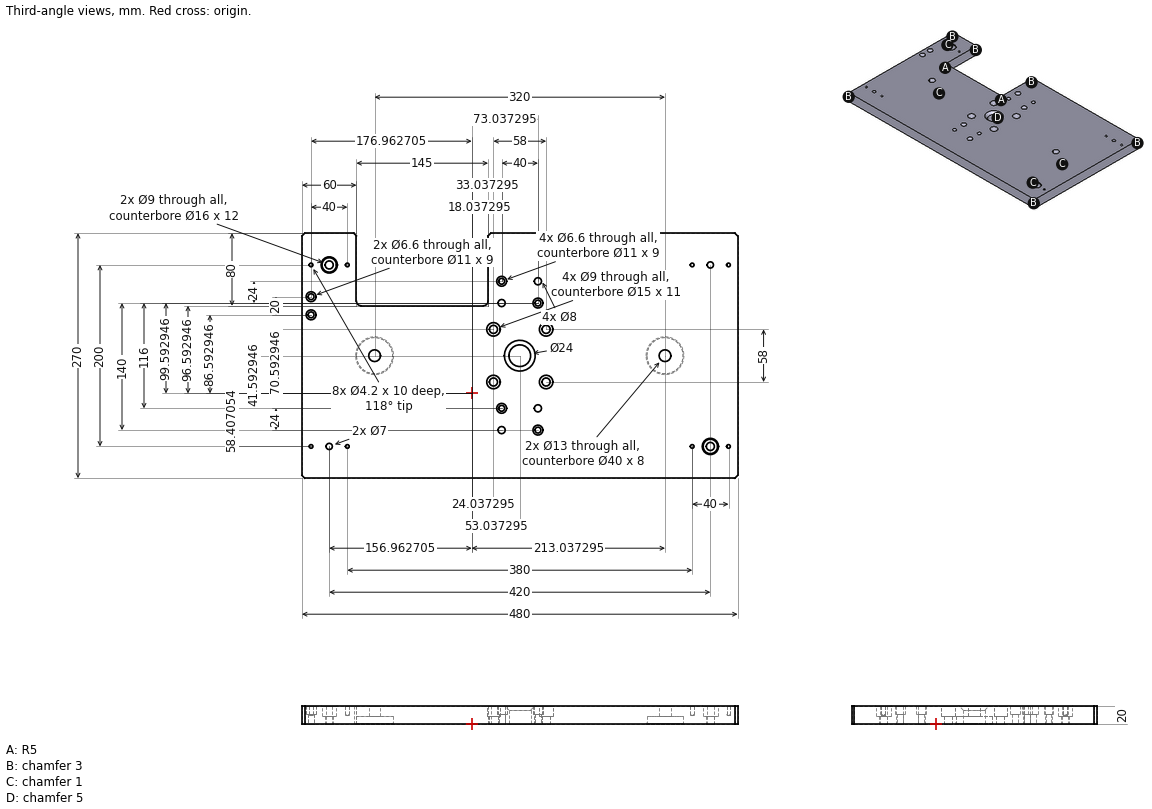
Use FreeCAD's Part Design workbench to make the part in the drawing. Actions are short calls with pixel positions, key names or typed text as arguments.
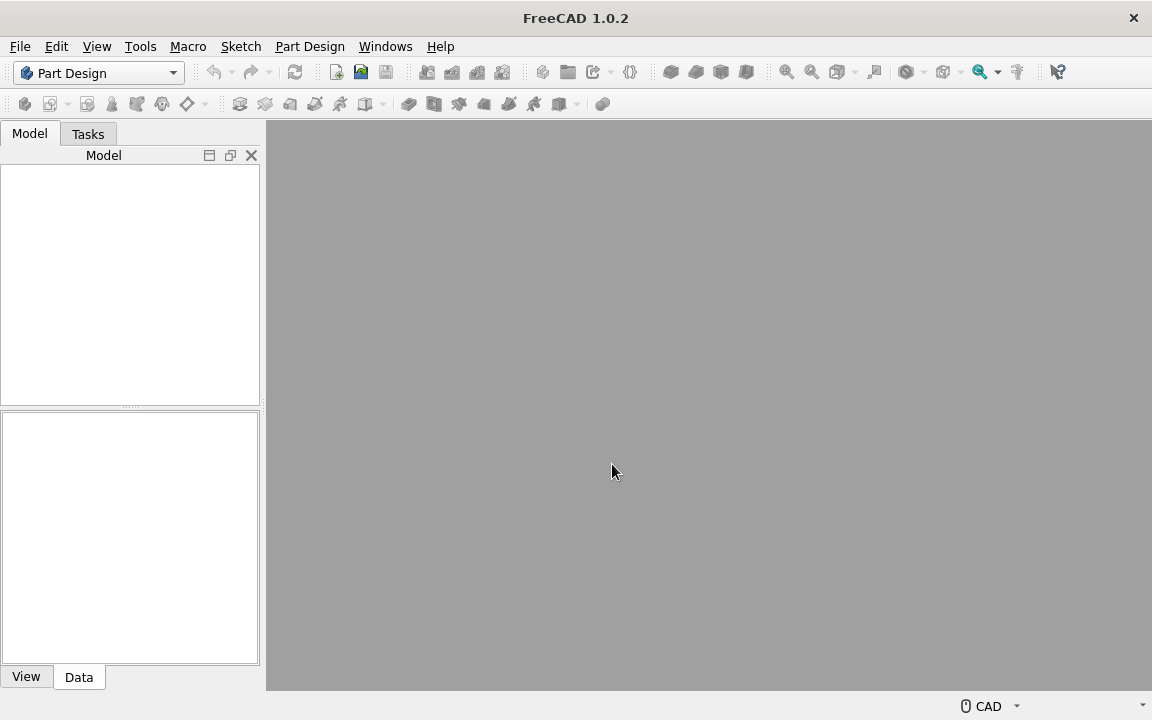
click(336, 72)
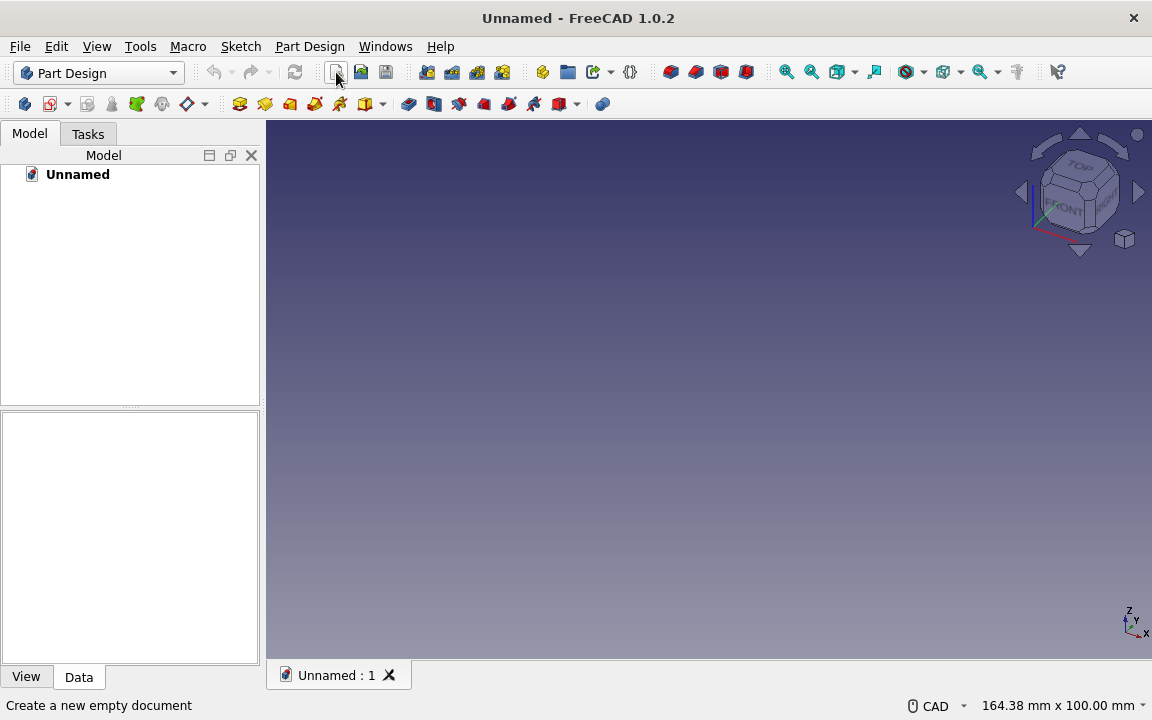
click(50, 104)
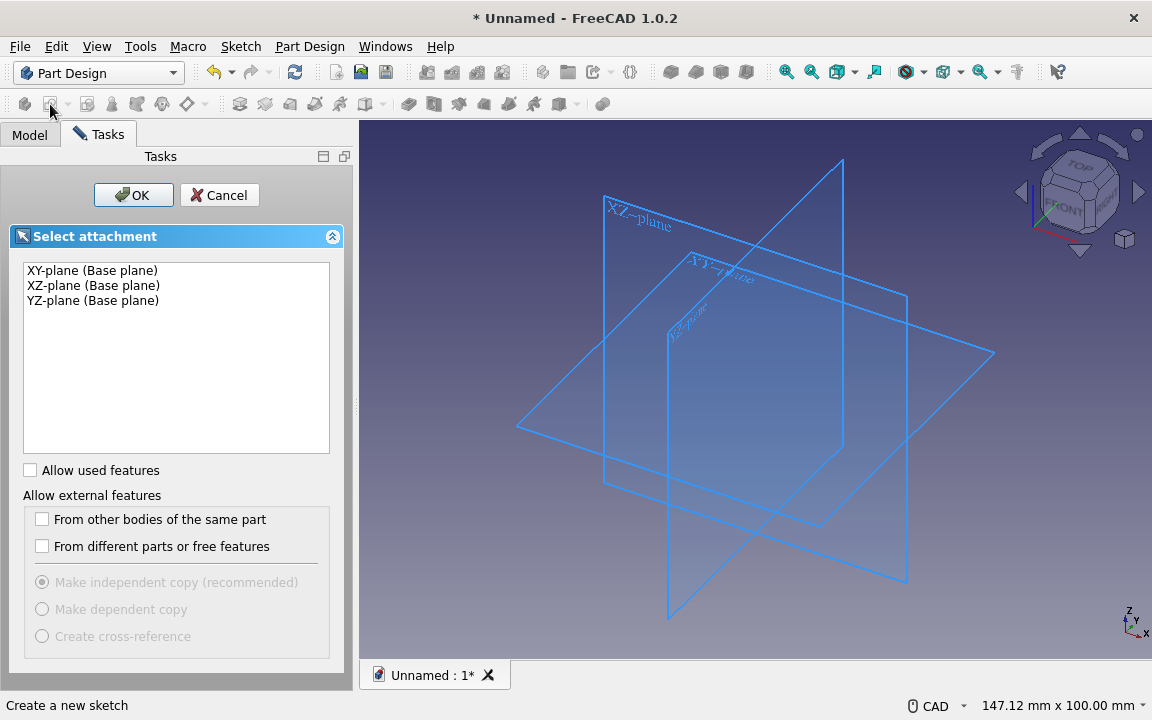
click(84, 270)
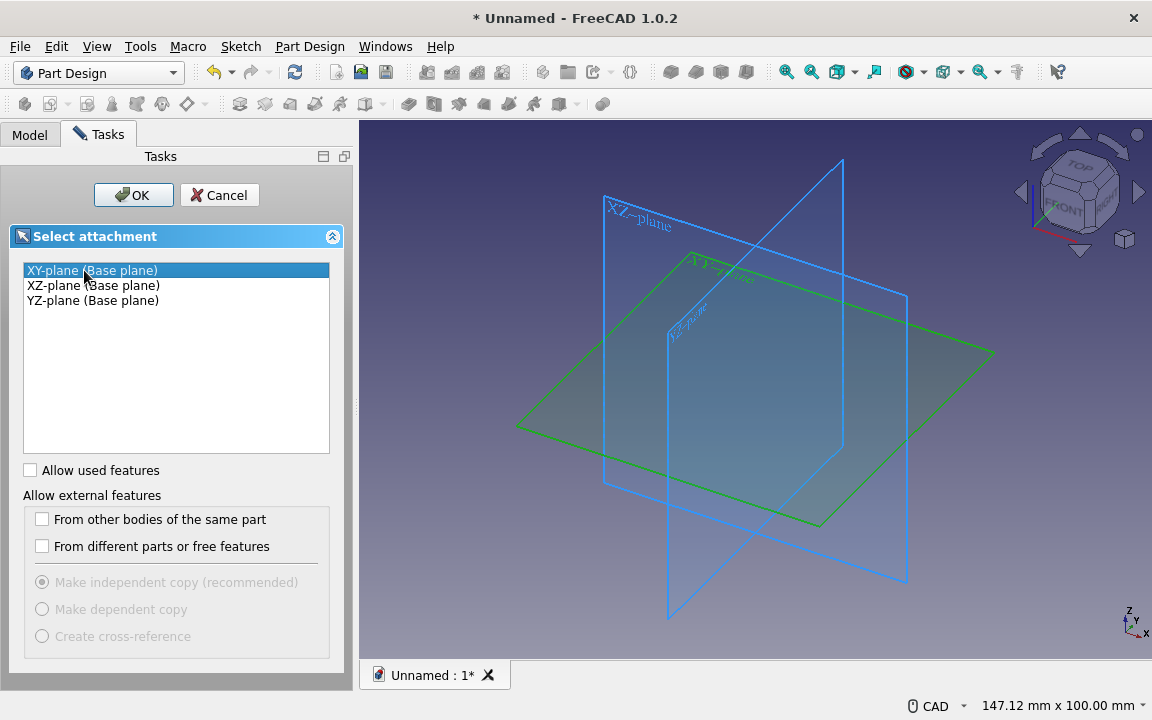
click(134, 195)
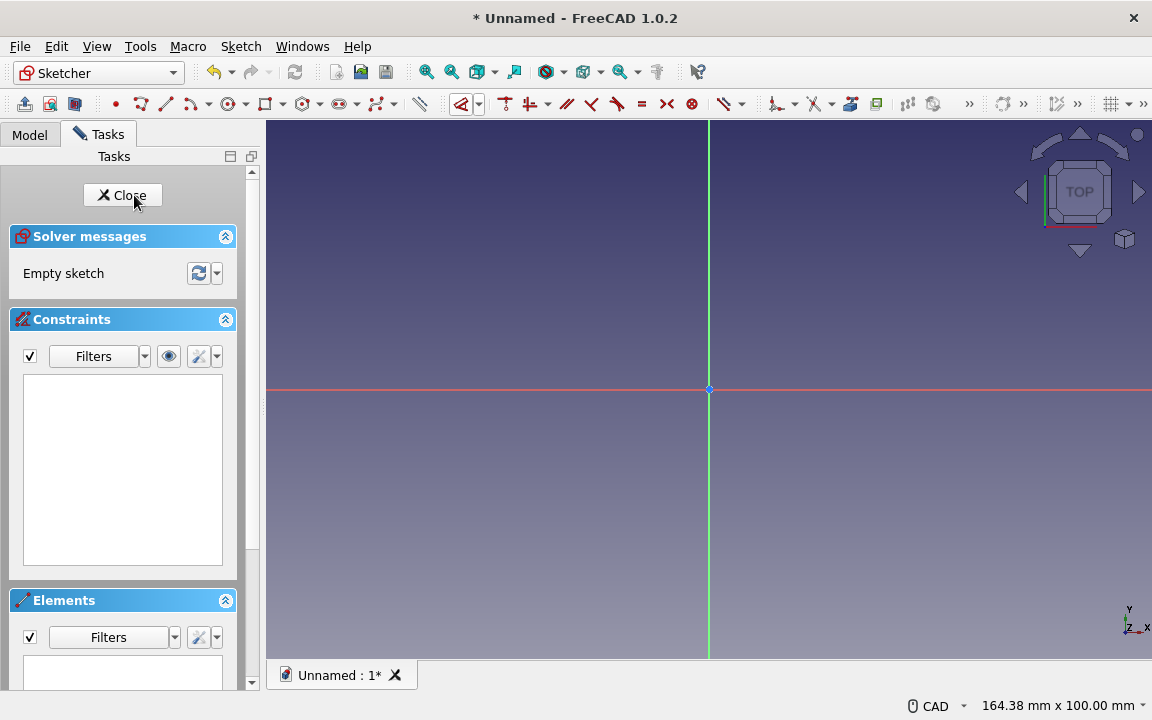
scroll(551, 446, down, 8)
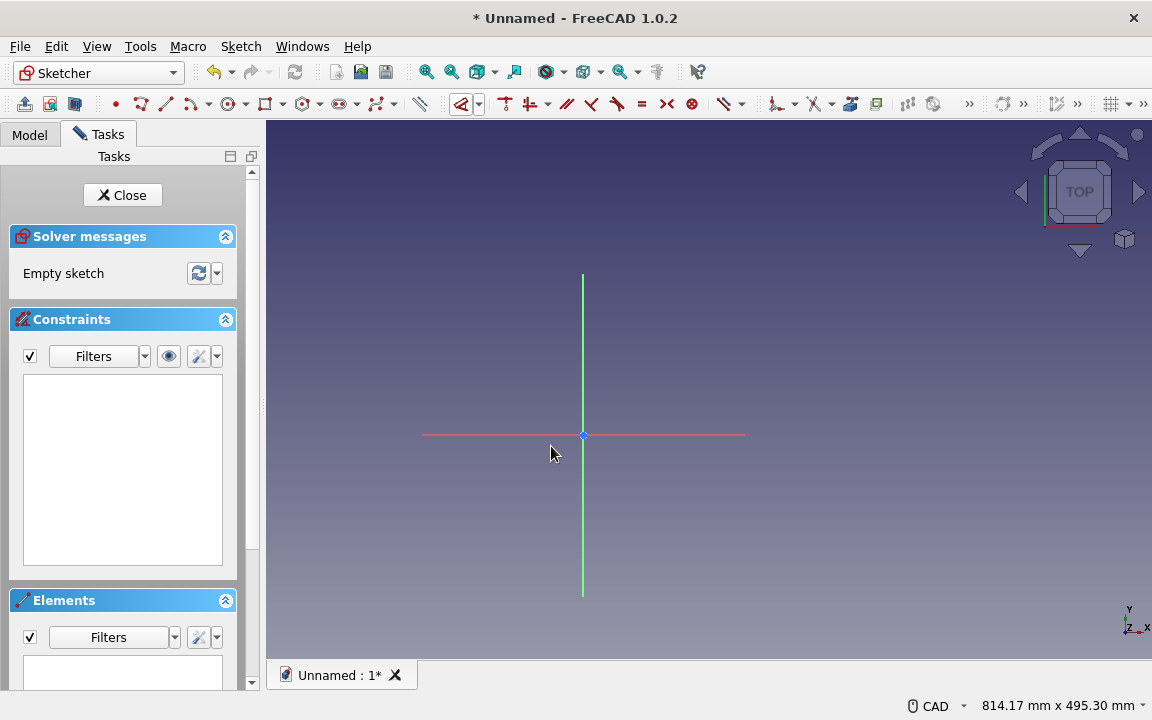
key(g)
key(m)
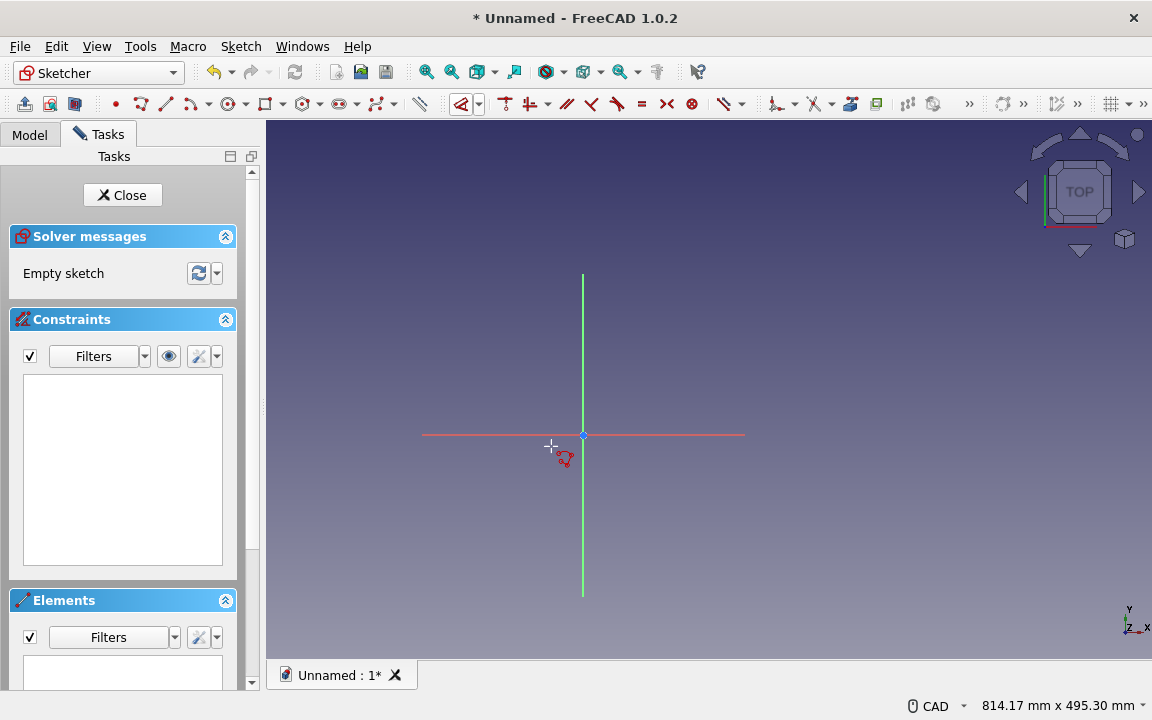
click(603, 330)
click(445, 330)
click(445, 243)
click(380, 243)
click(380, 537)
click(902, 537)
click(902, 243)
click(603, 243)
click(603, 331)
key(Escape)
key(Escape)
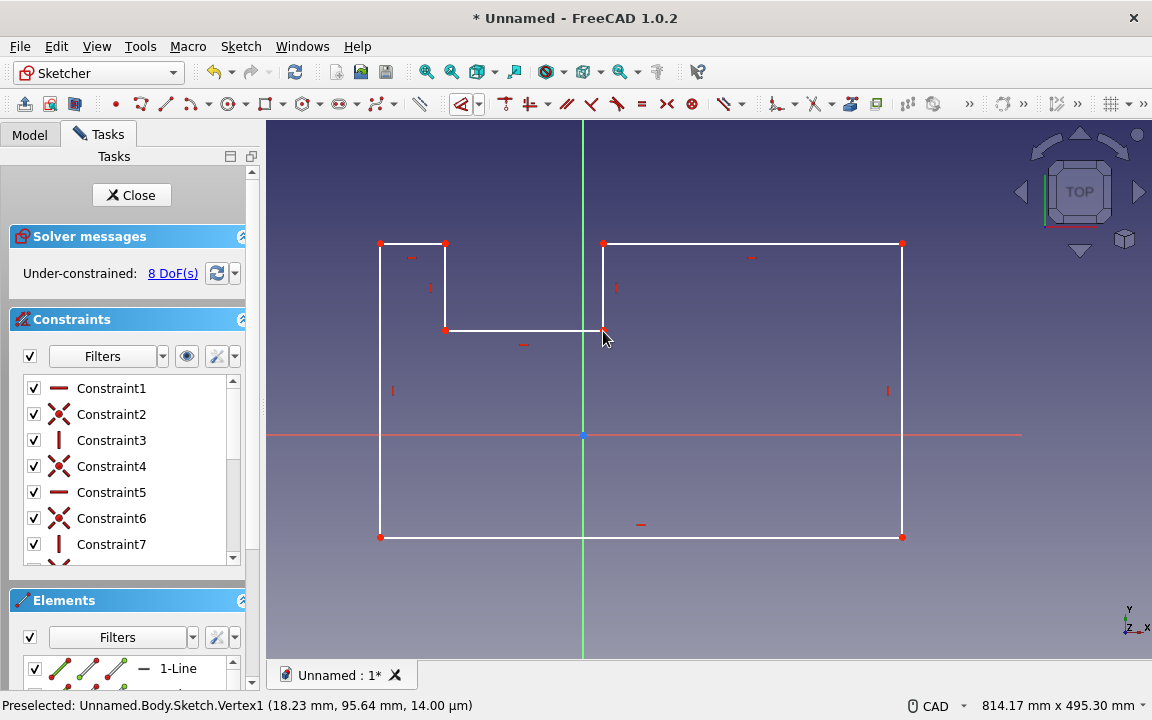
click(460, 104)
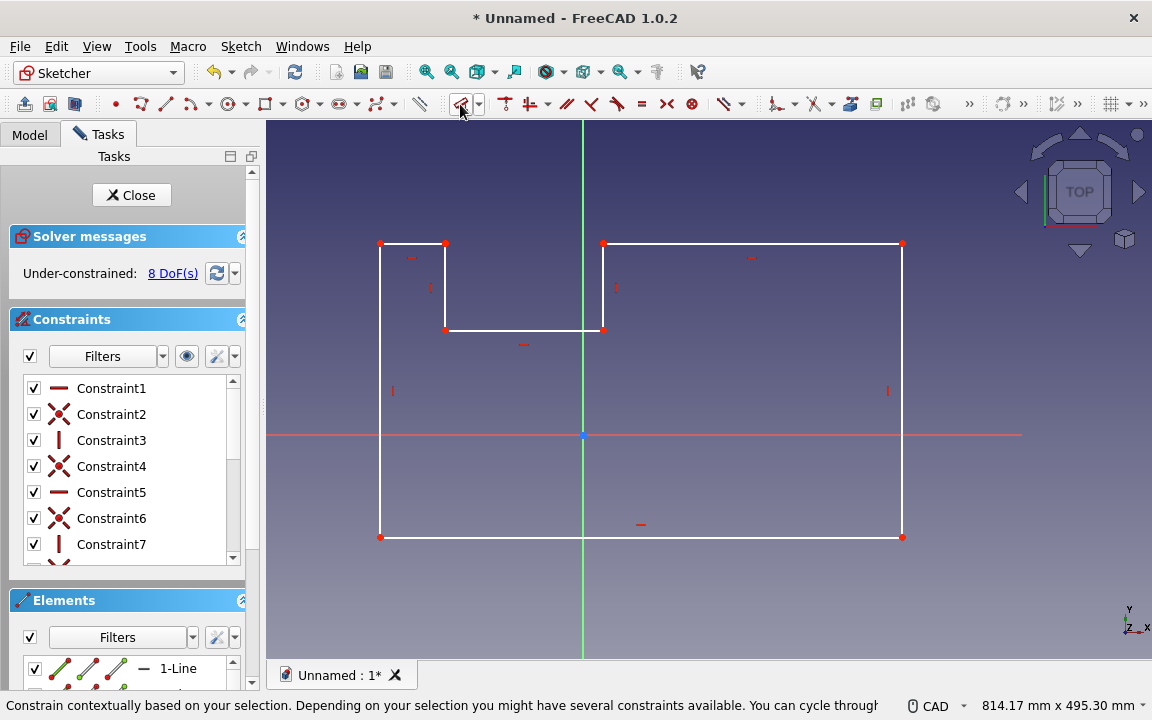
click(445, 305)
click(411, 287)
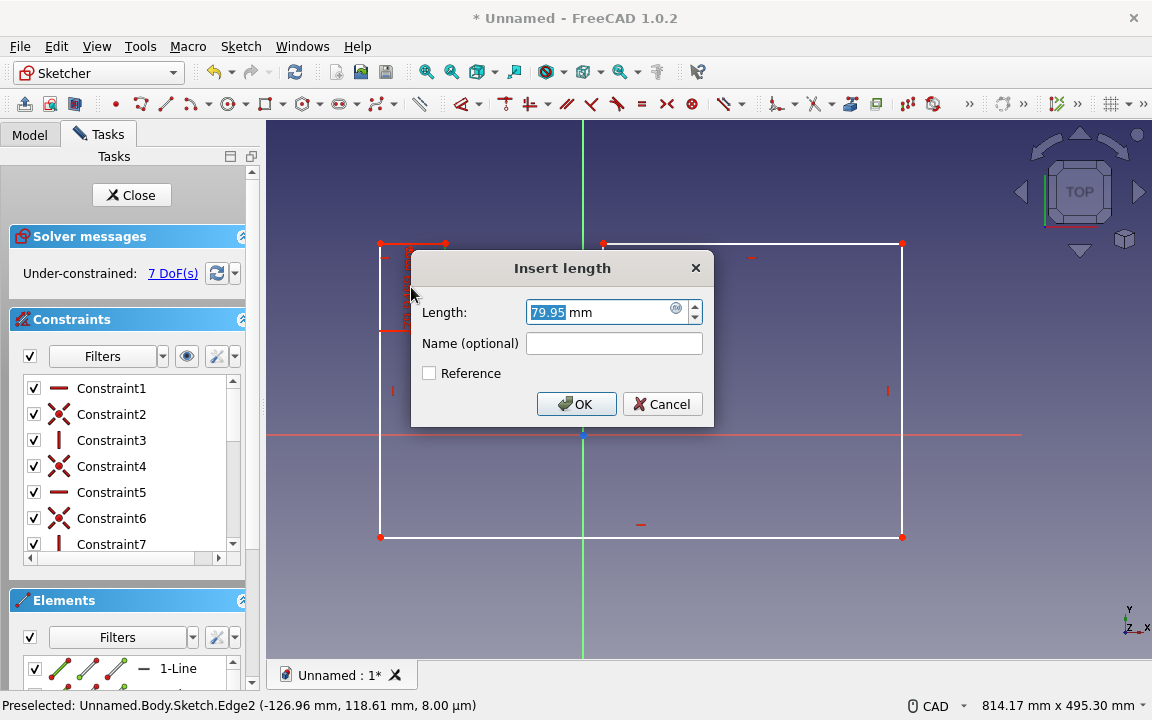
text(80)
key(Return)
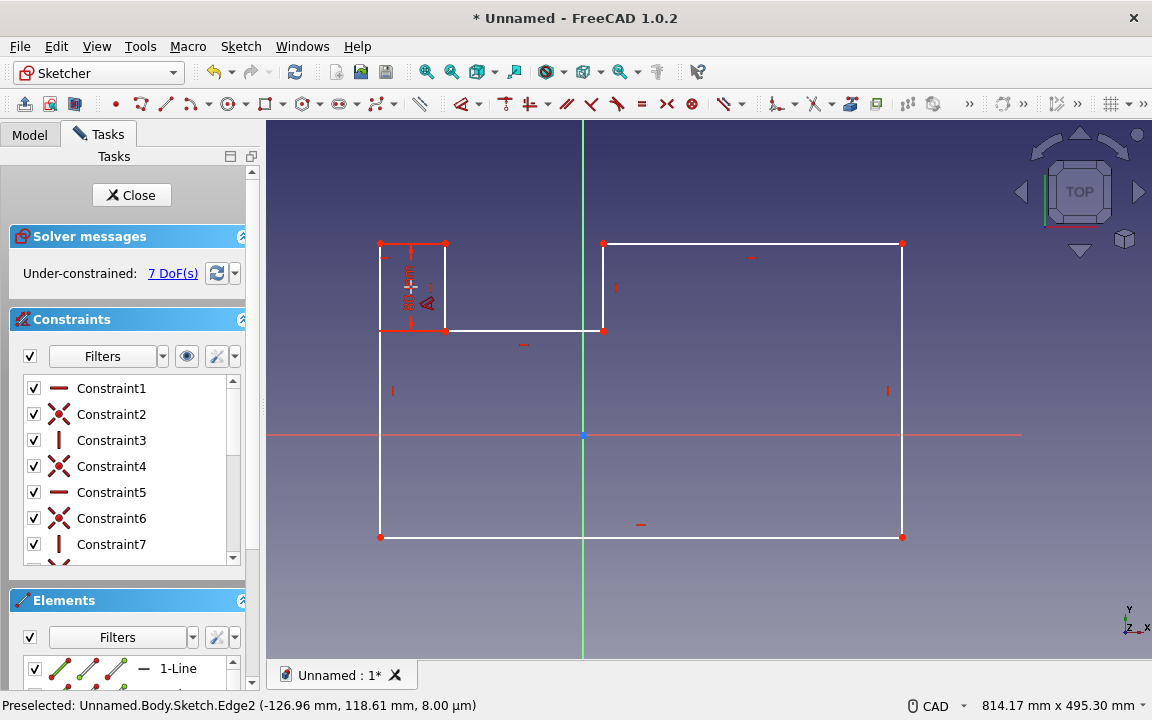
click(426, 244)
click(413, 210)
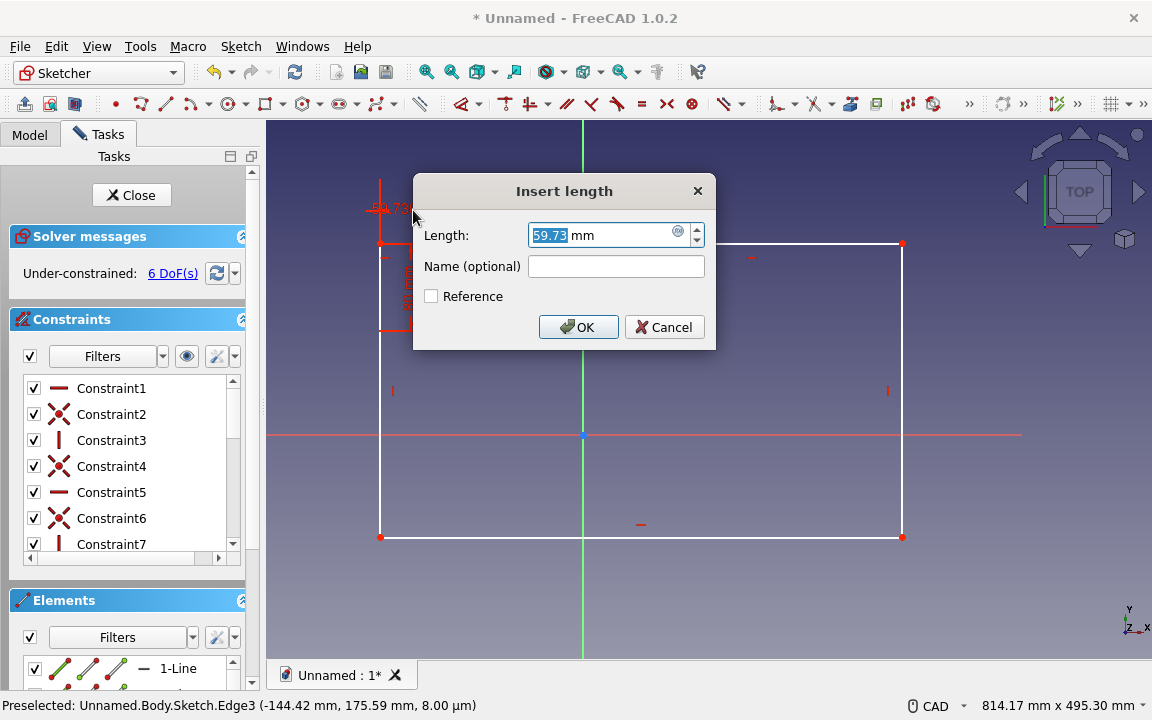
text(60)
key(Return)